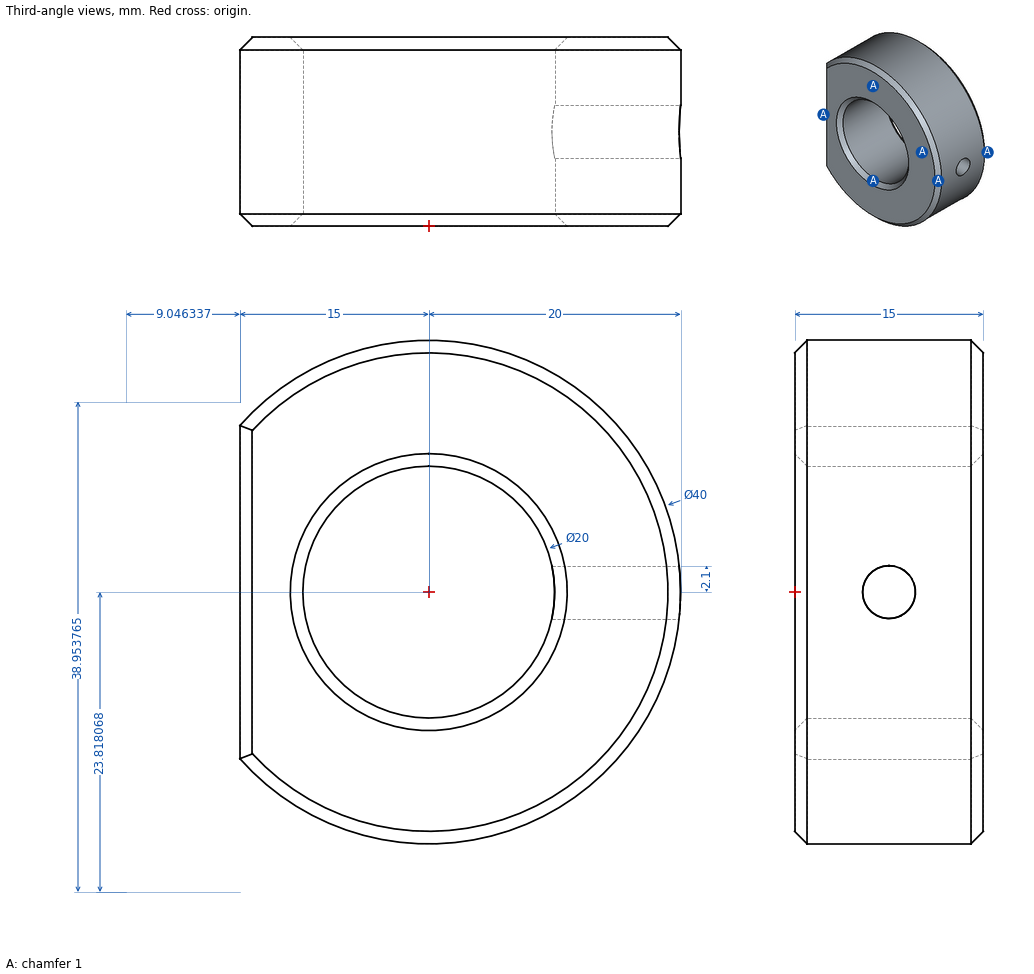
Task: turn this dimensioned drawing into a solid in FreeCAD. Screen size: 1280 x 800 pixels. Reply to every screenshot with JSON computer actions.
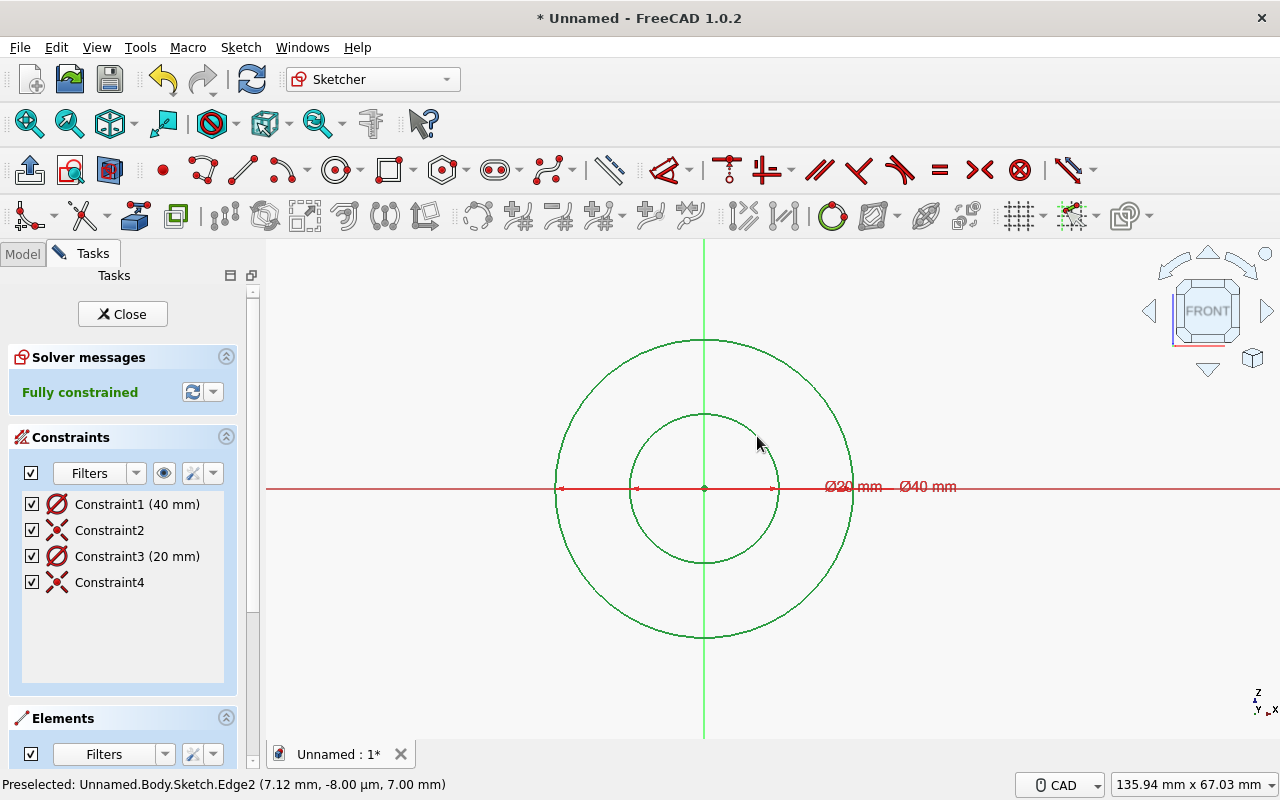
{"action": "left_click", "coordinate": [123, 314]}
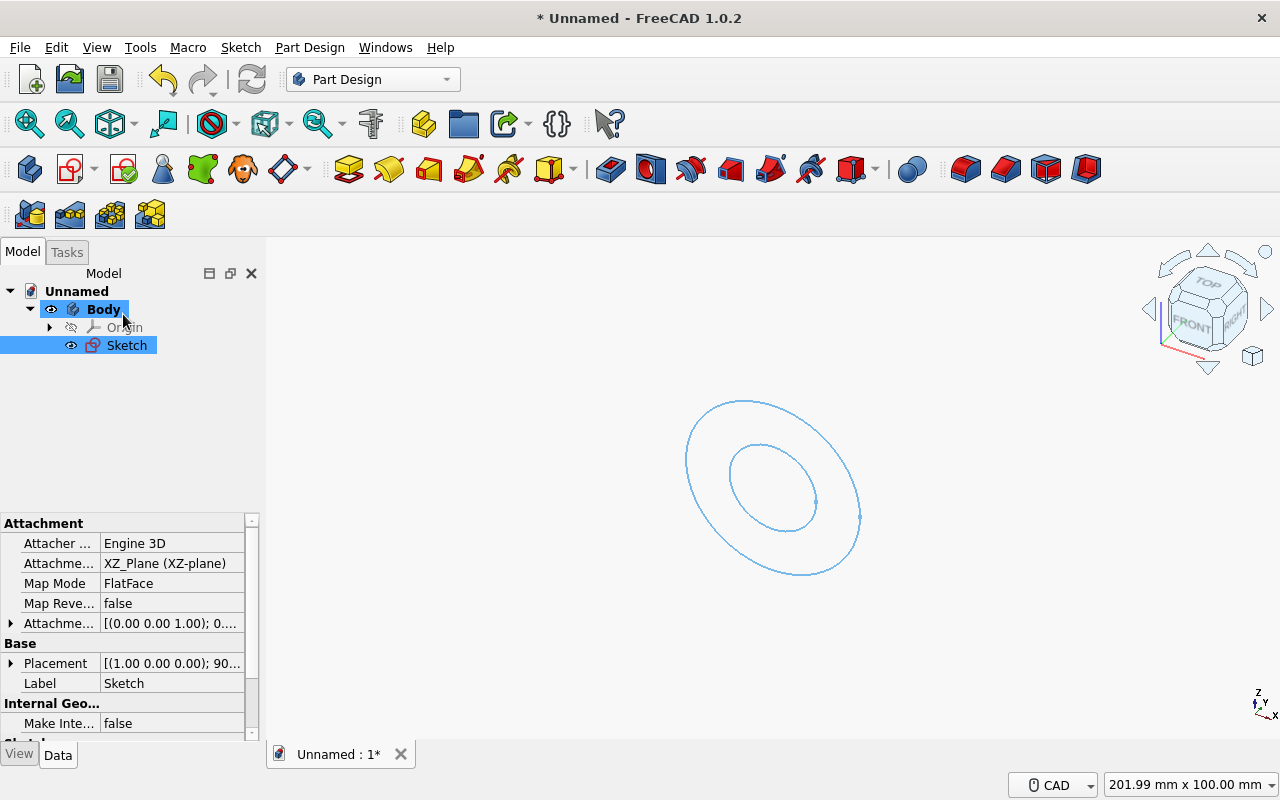
{"action": "left_click", "coordinate": [350, 170]}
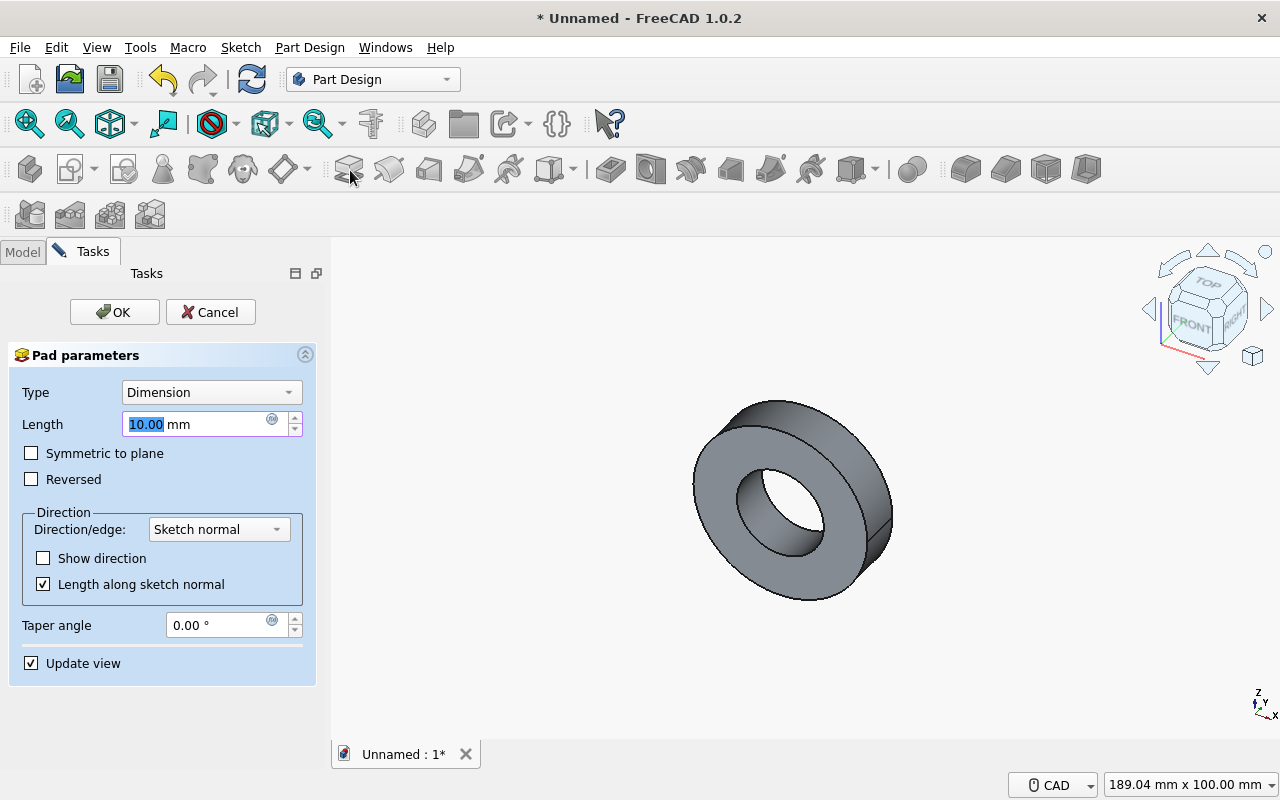
{"action": "type", "text": "15"}
{"action": "key", "text": "Tab"}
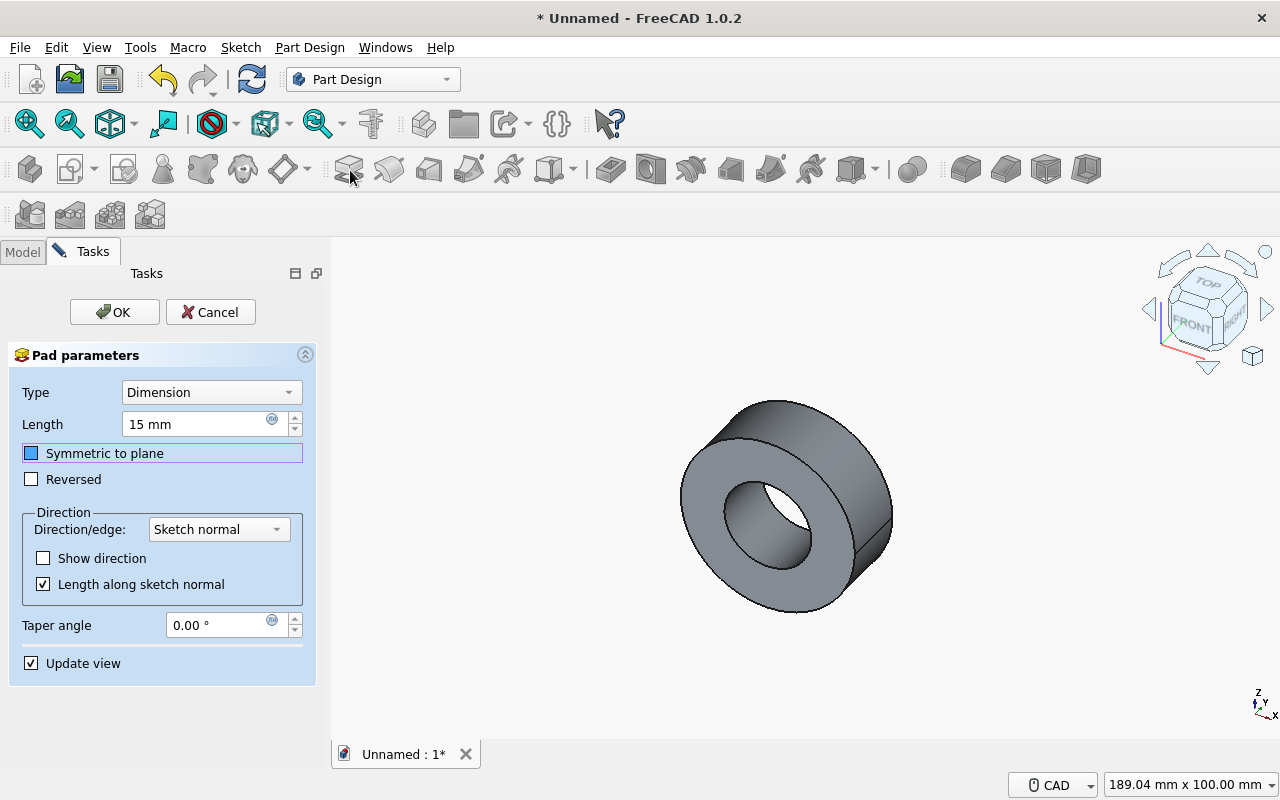
{"action": "left_click", "coordinate": [30, 479]}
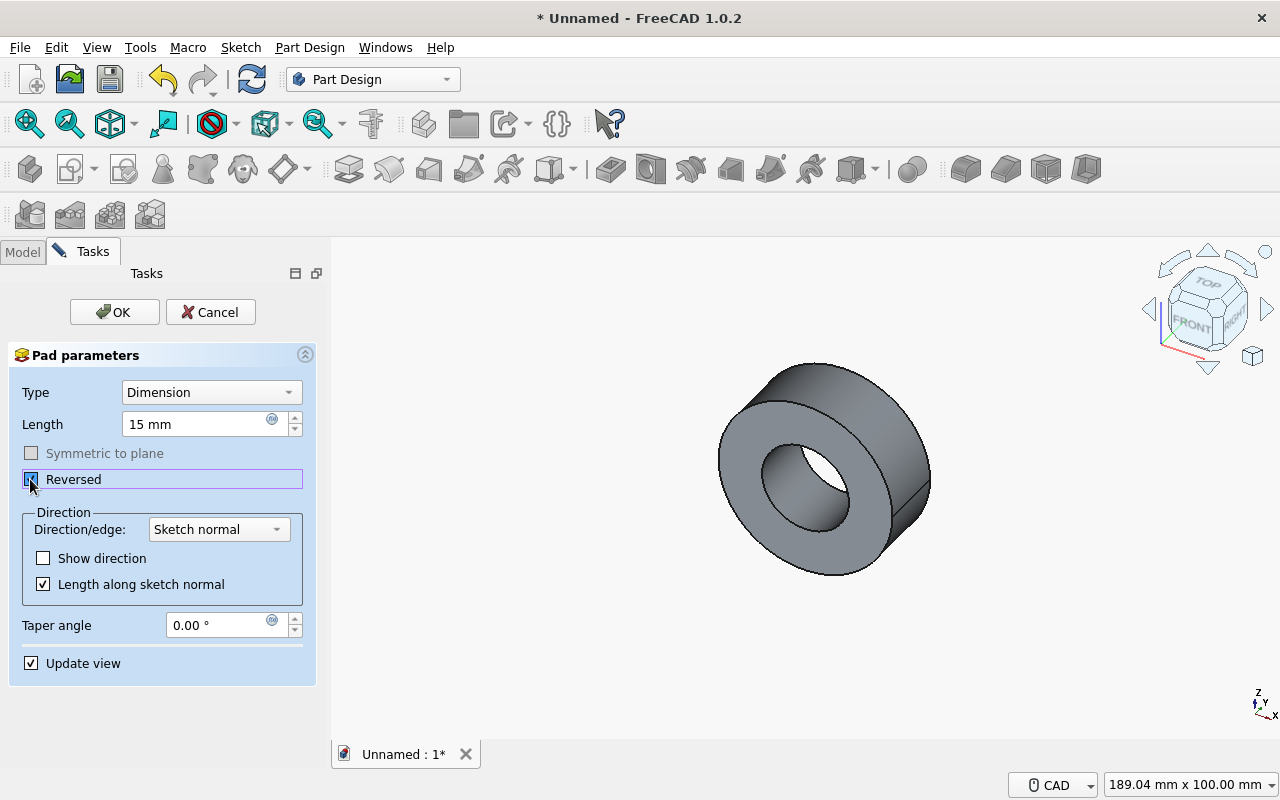
{"action": "left_click", "coordinate": [115, 312]}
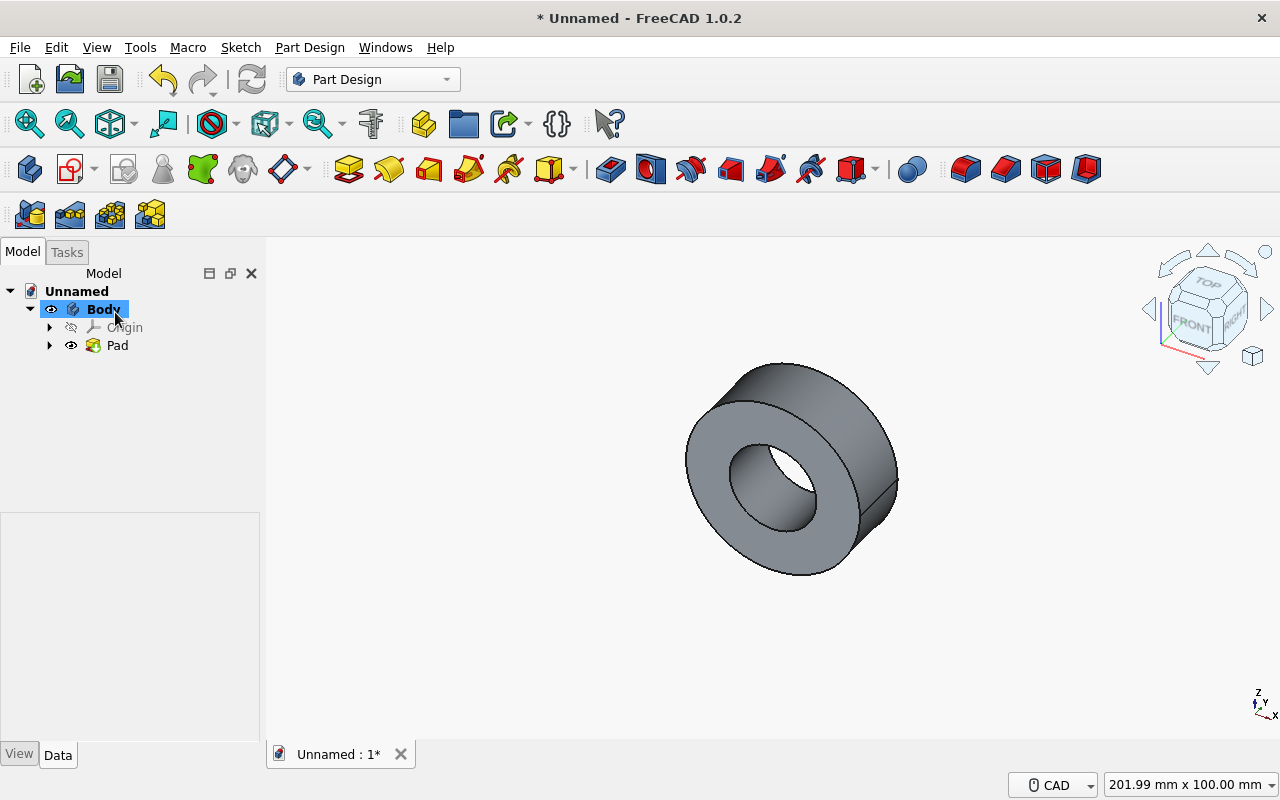
{"action": "key", "text": "4"}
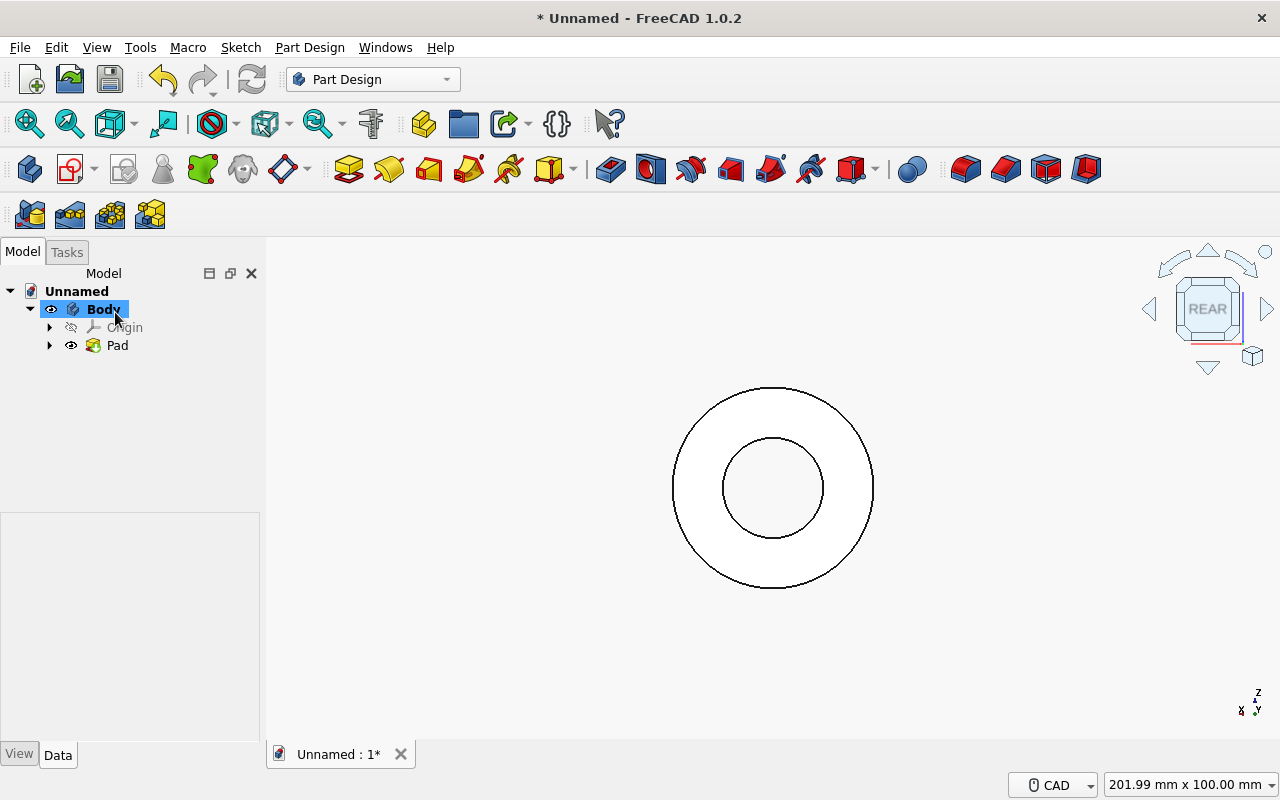
{"action": "left_click", "coordinate": [30, 124]}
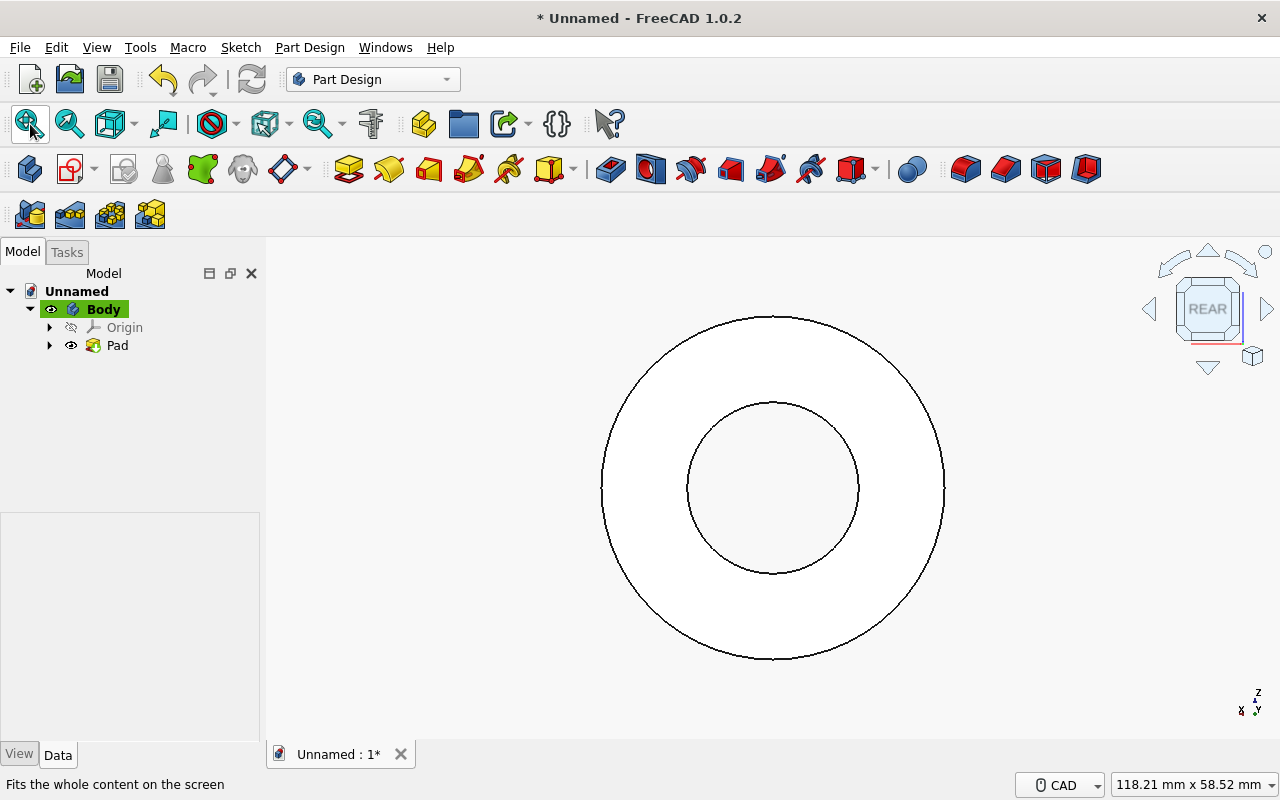
{"action": "left_click", "coordinate": [675, 585]}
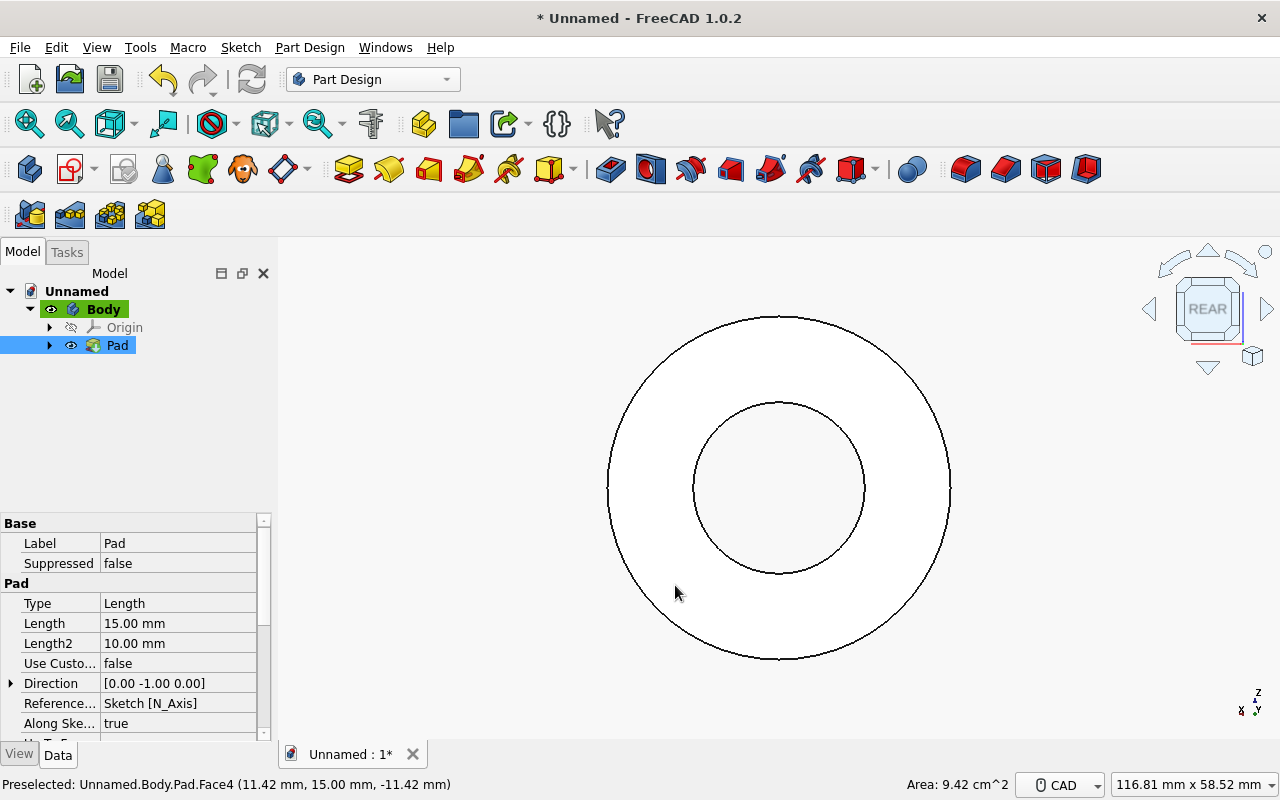
{"action": "left_click", "coordinate": [70, 170]}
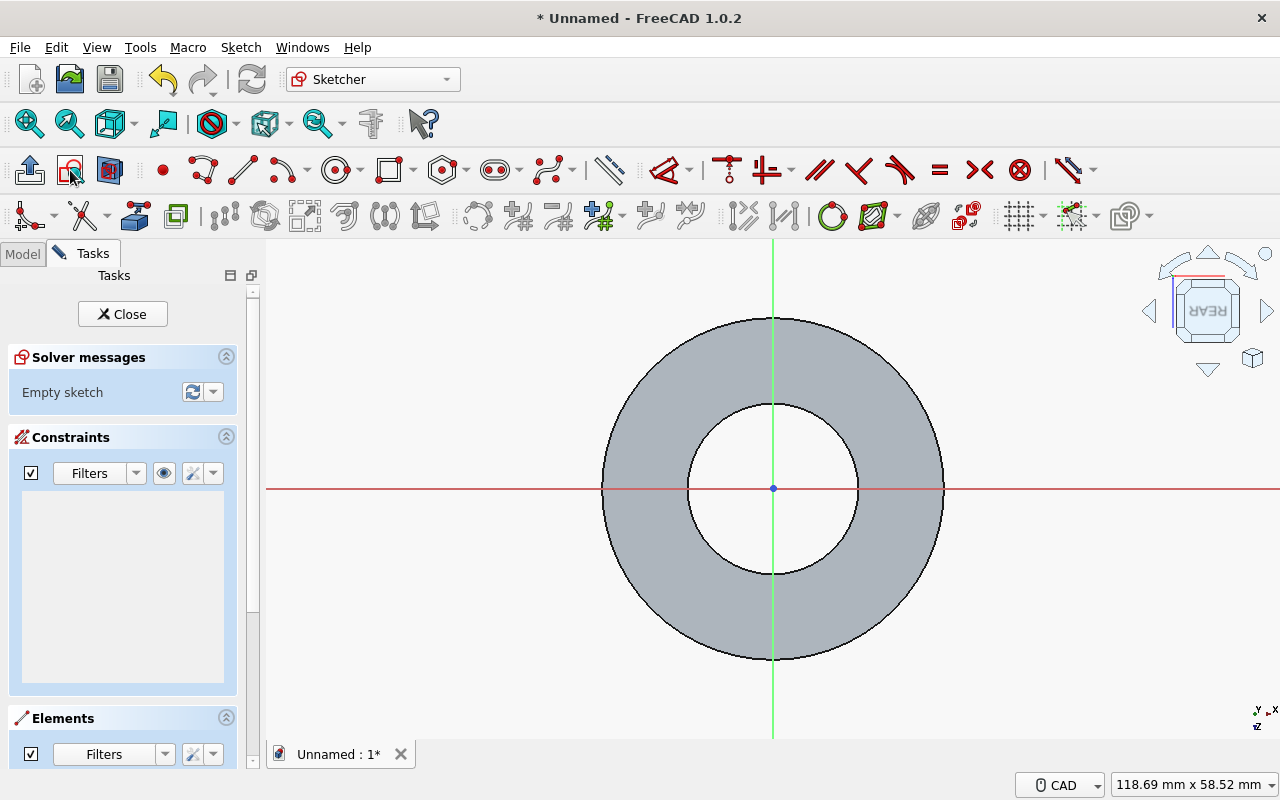
{"action": "scroll", "coordinate": [859, 657], "scroll_direction": "down", "scroll_amount": 1}